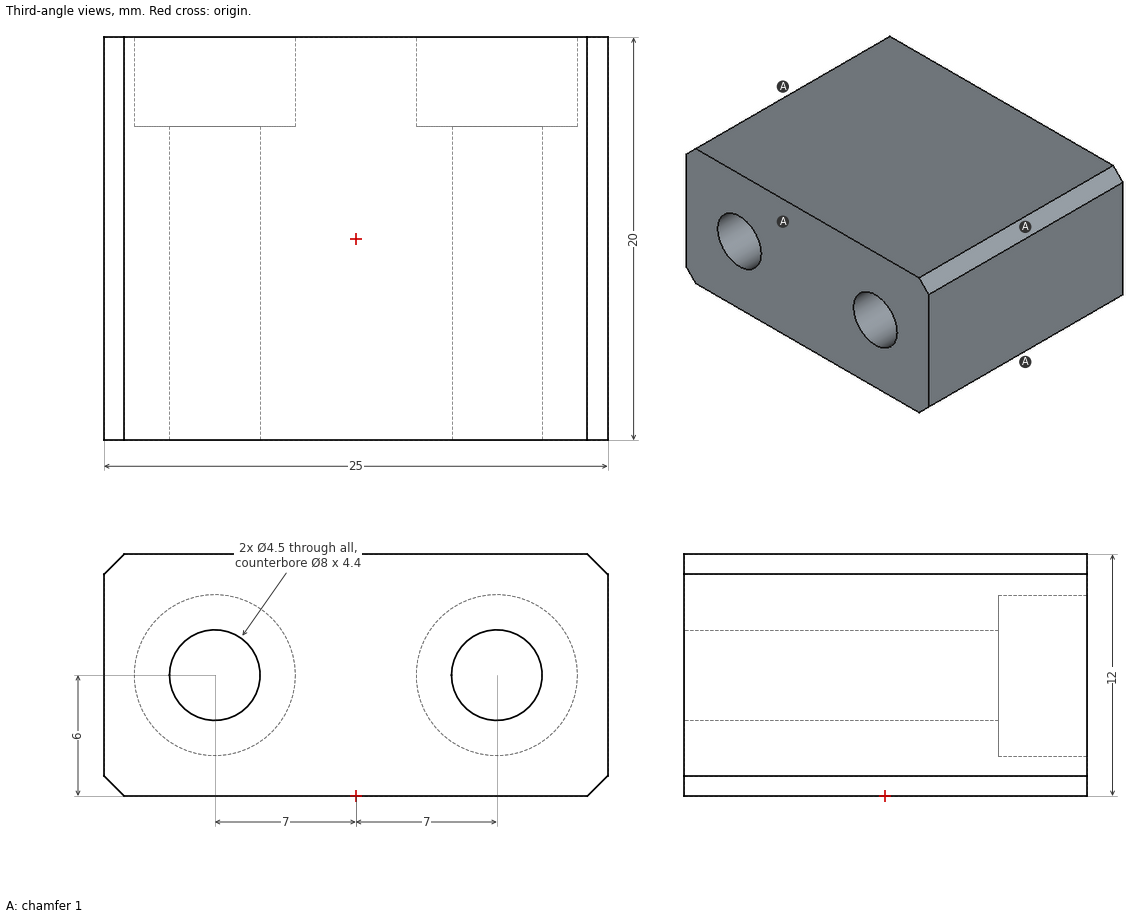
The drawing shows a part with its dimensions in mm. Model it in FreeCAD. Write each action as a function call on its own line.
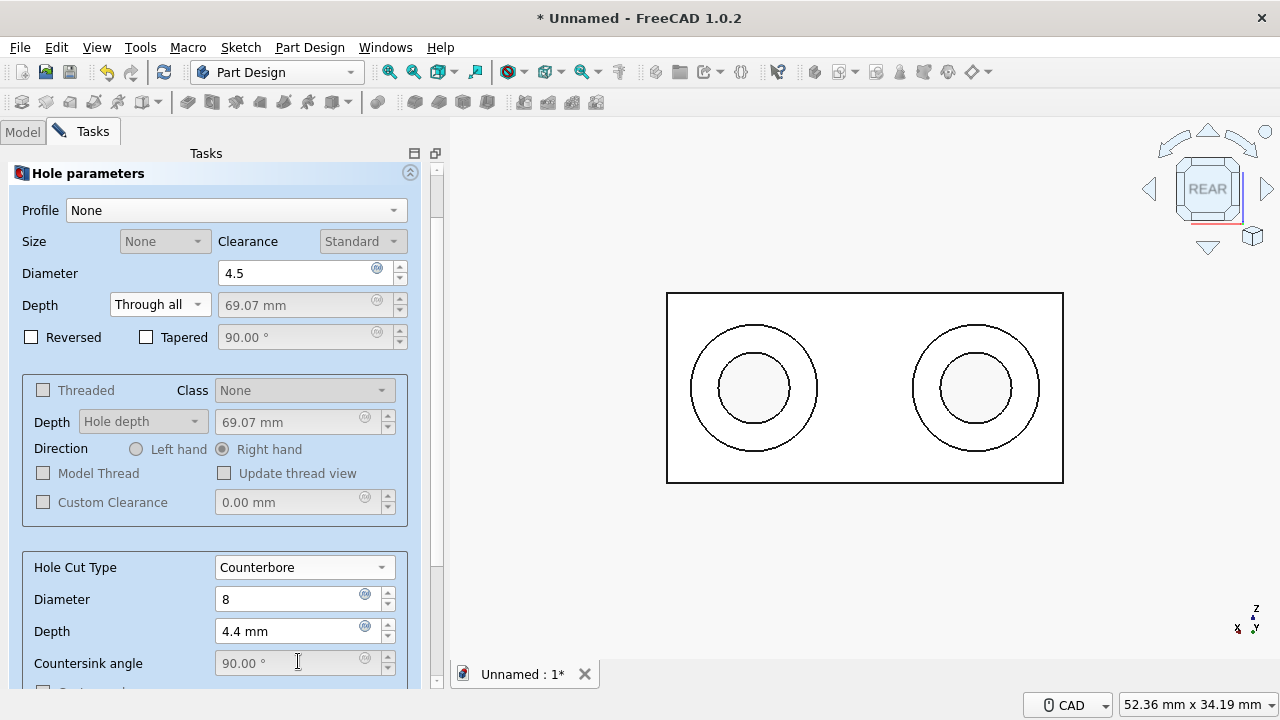
scroll(437, 426, up, 2)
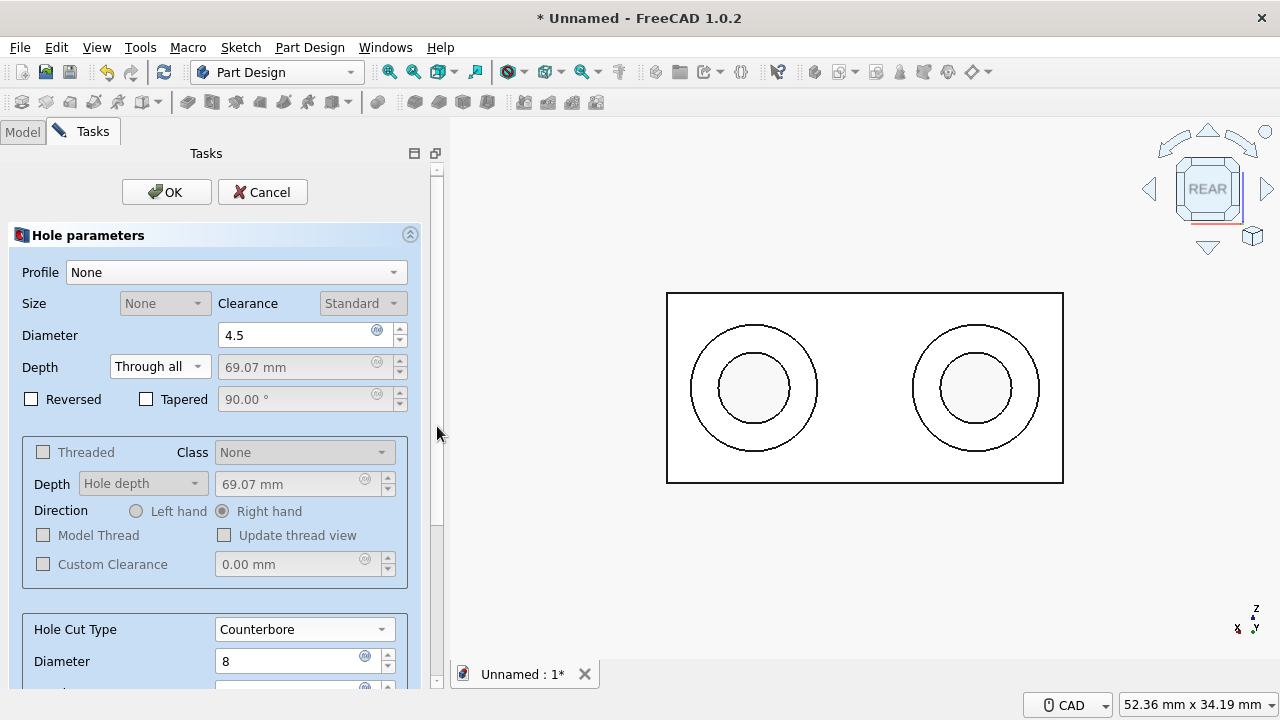
click(167, 192)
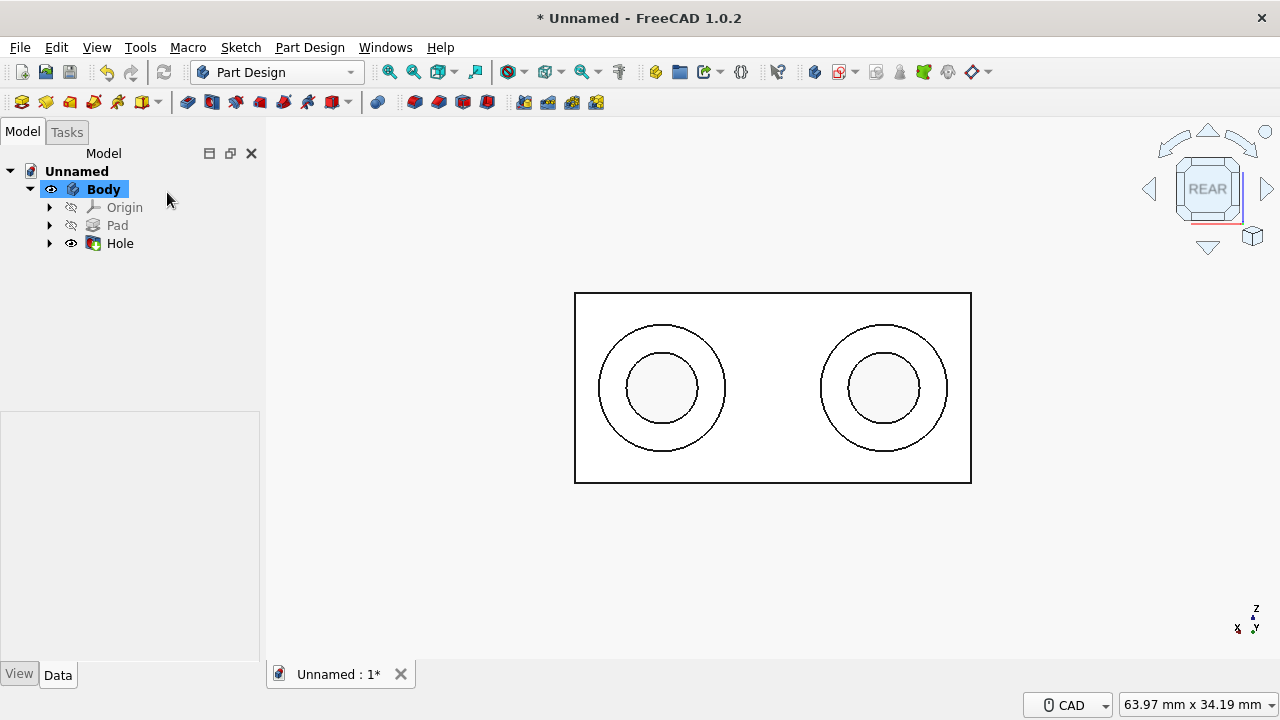
key(v)
key(f)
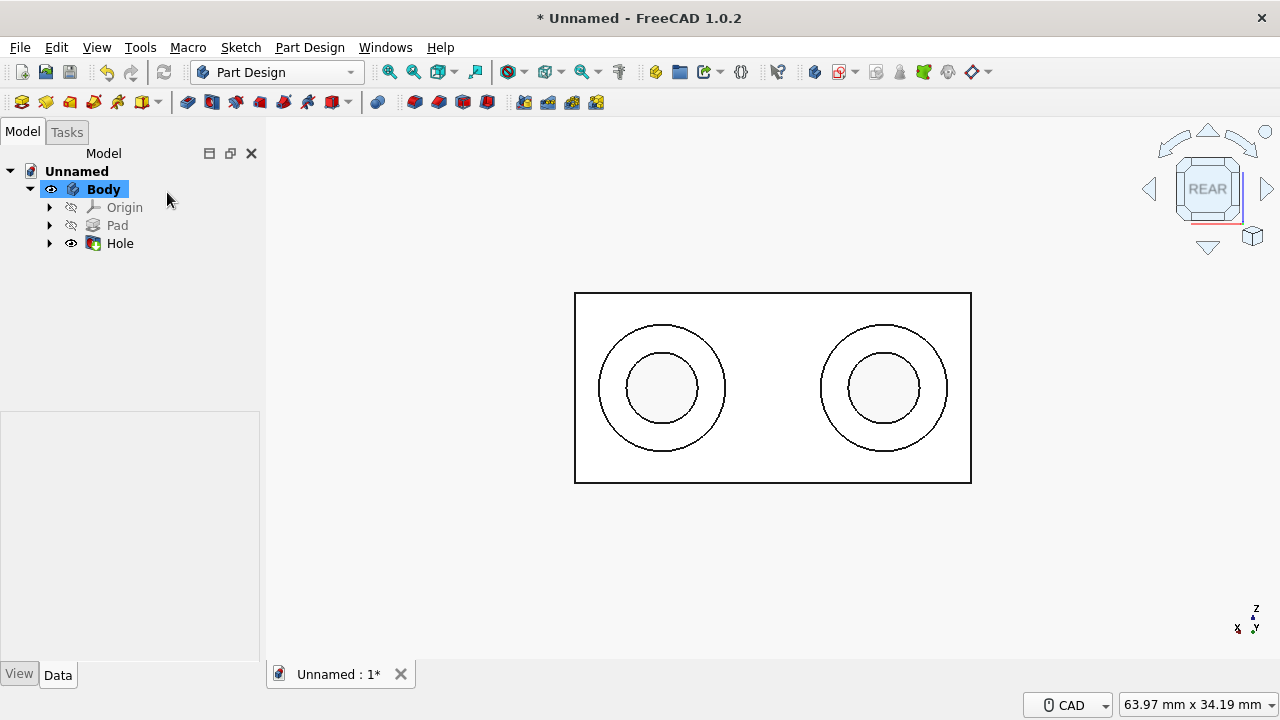
key(0)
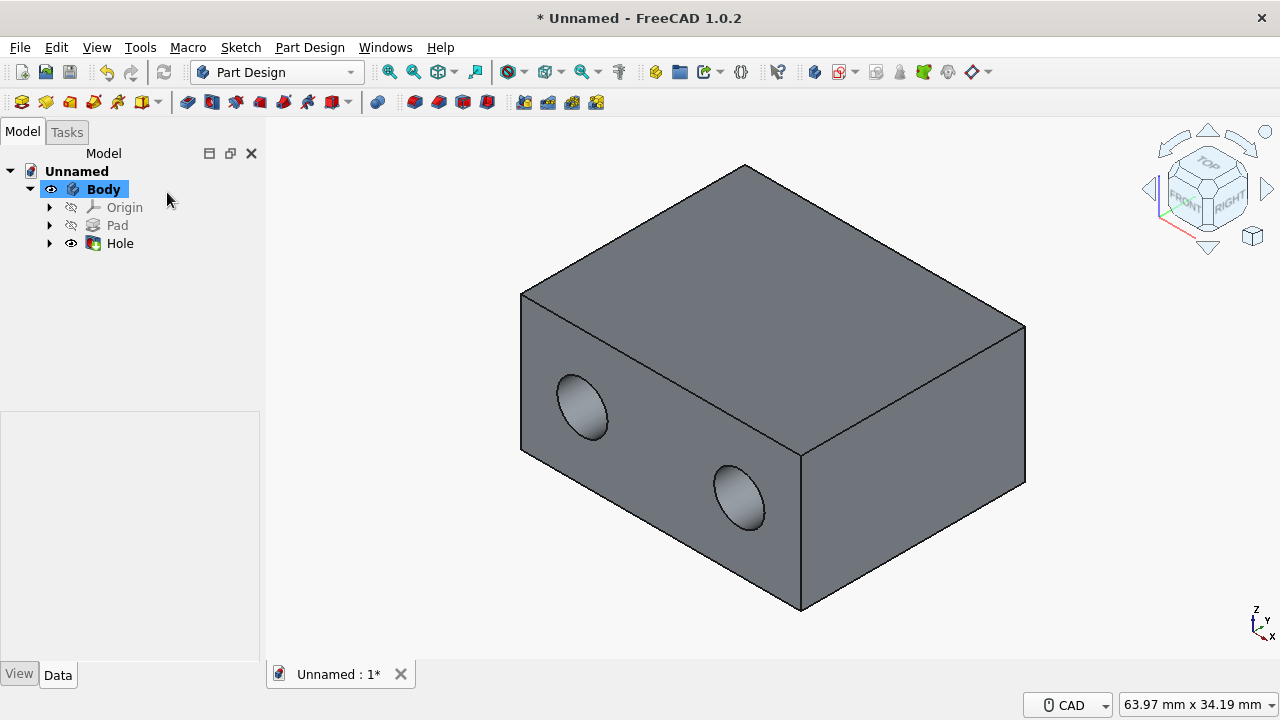
click(913, 390)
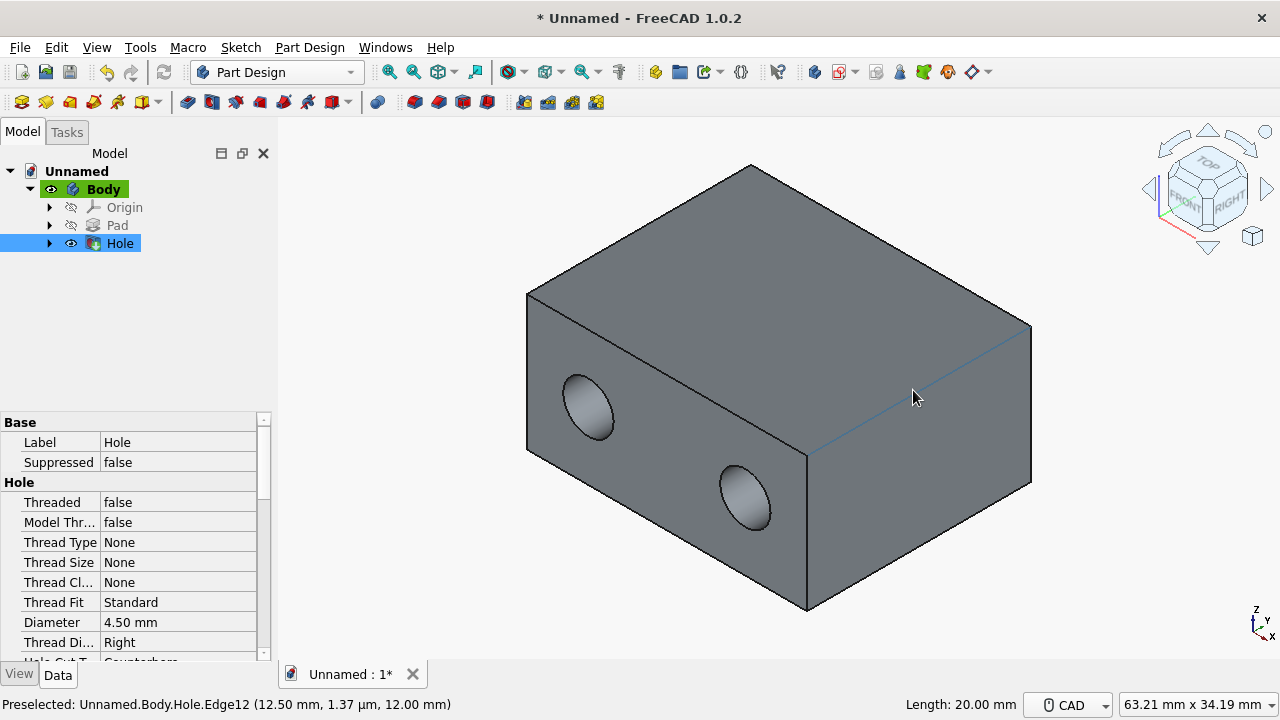
key(2)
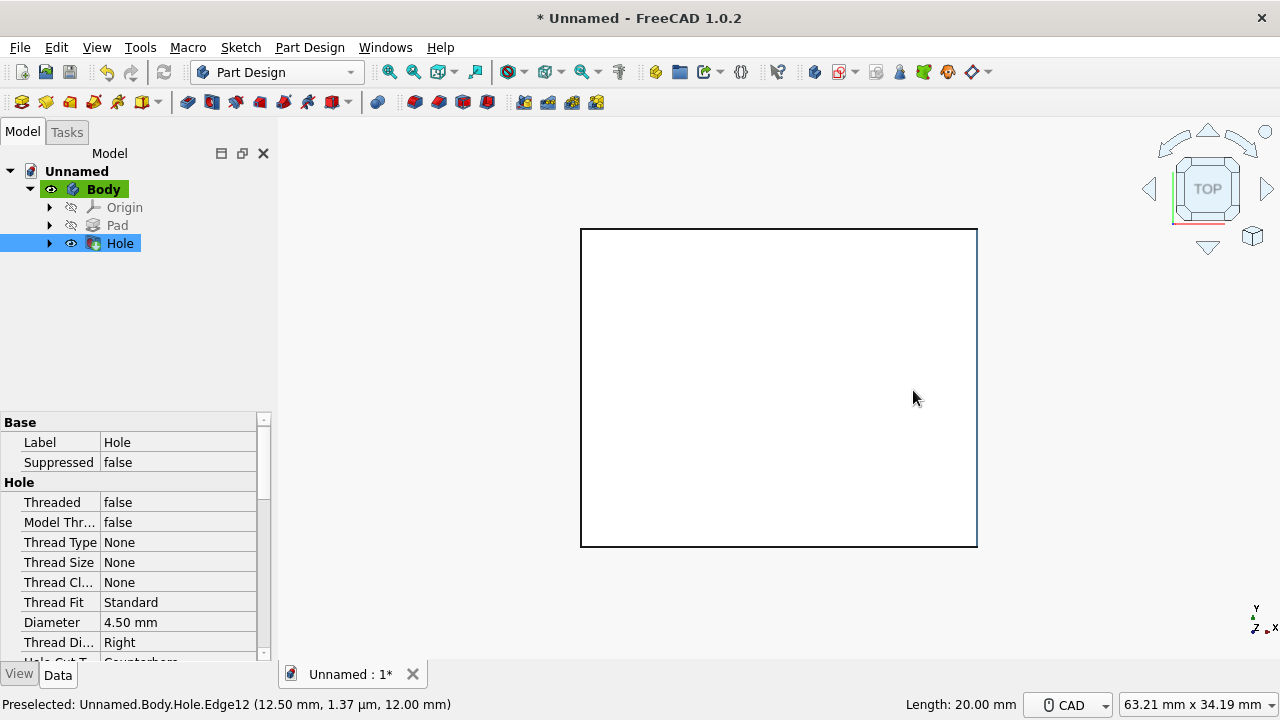
click(581, 387, ctrl)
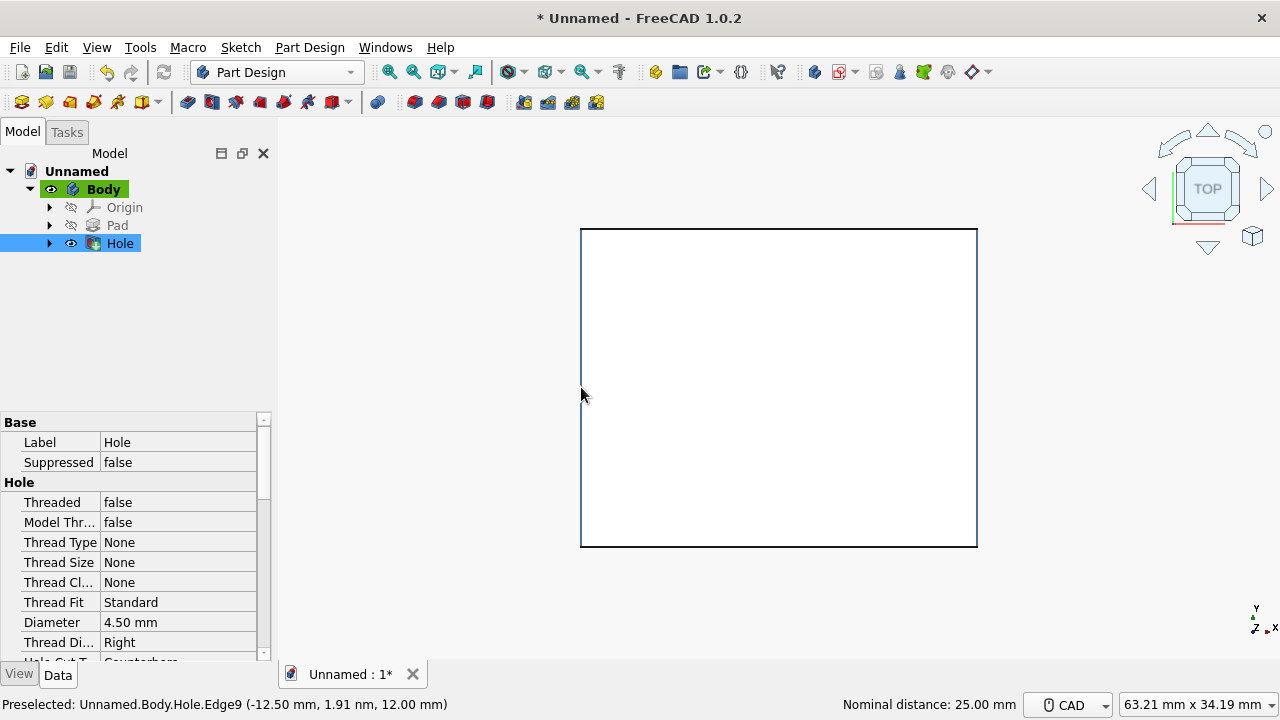
key(1)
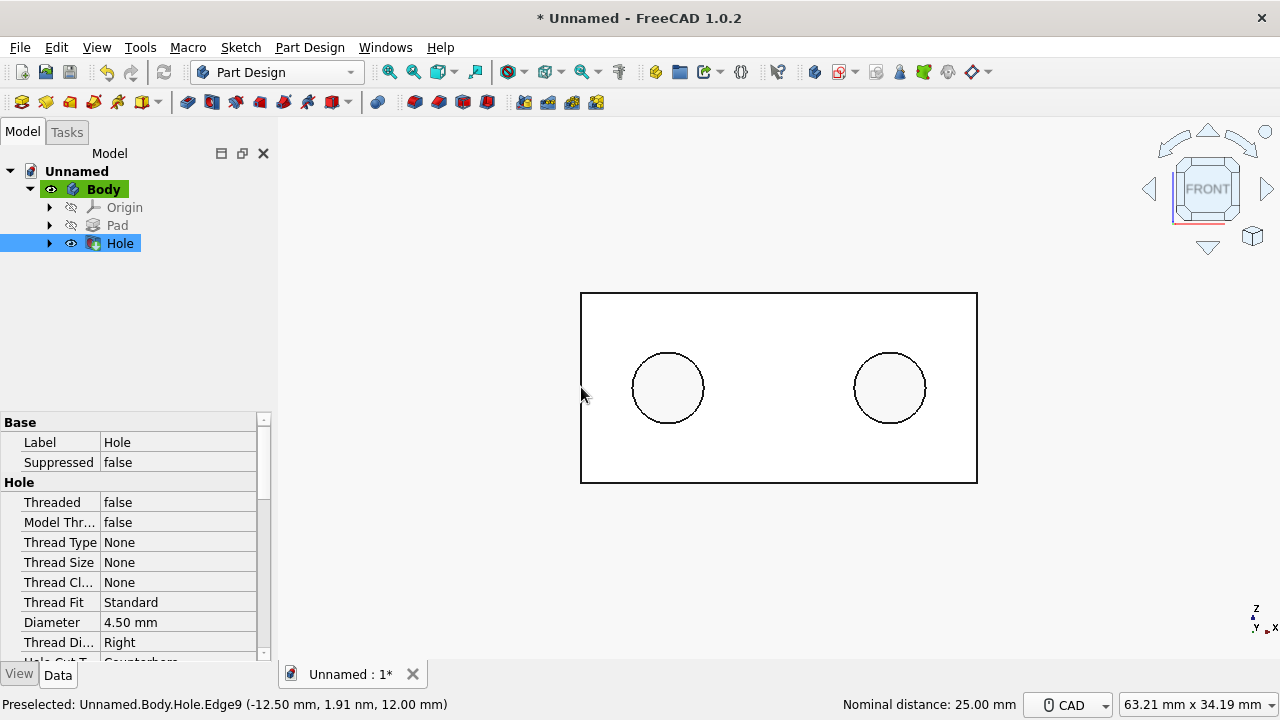
key(v)
key(f)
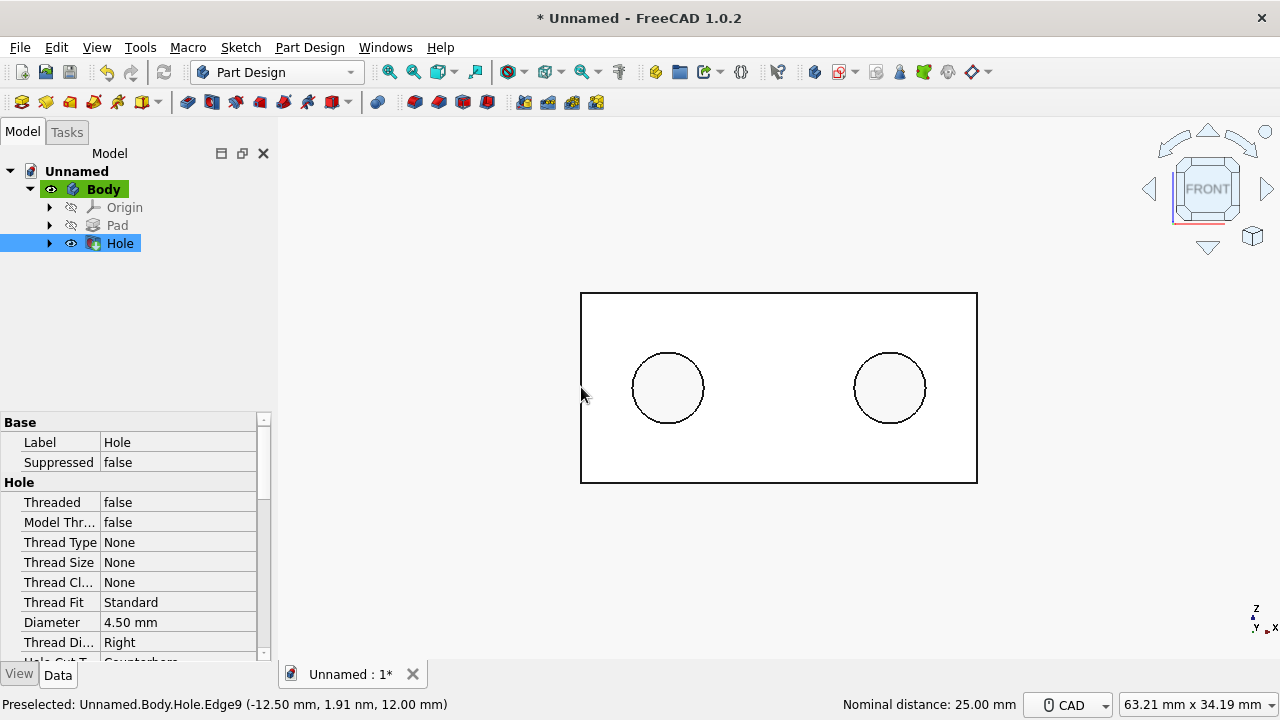
key(3)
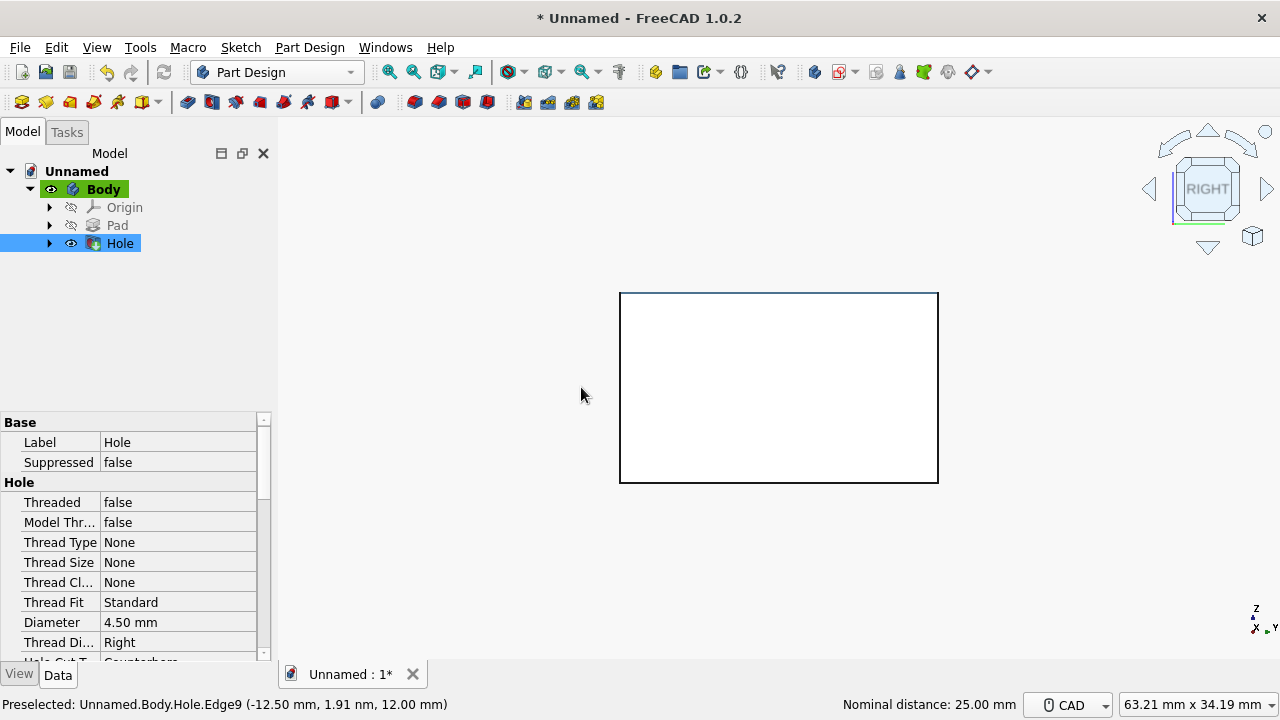
click(390, 72)